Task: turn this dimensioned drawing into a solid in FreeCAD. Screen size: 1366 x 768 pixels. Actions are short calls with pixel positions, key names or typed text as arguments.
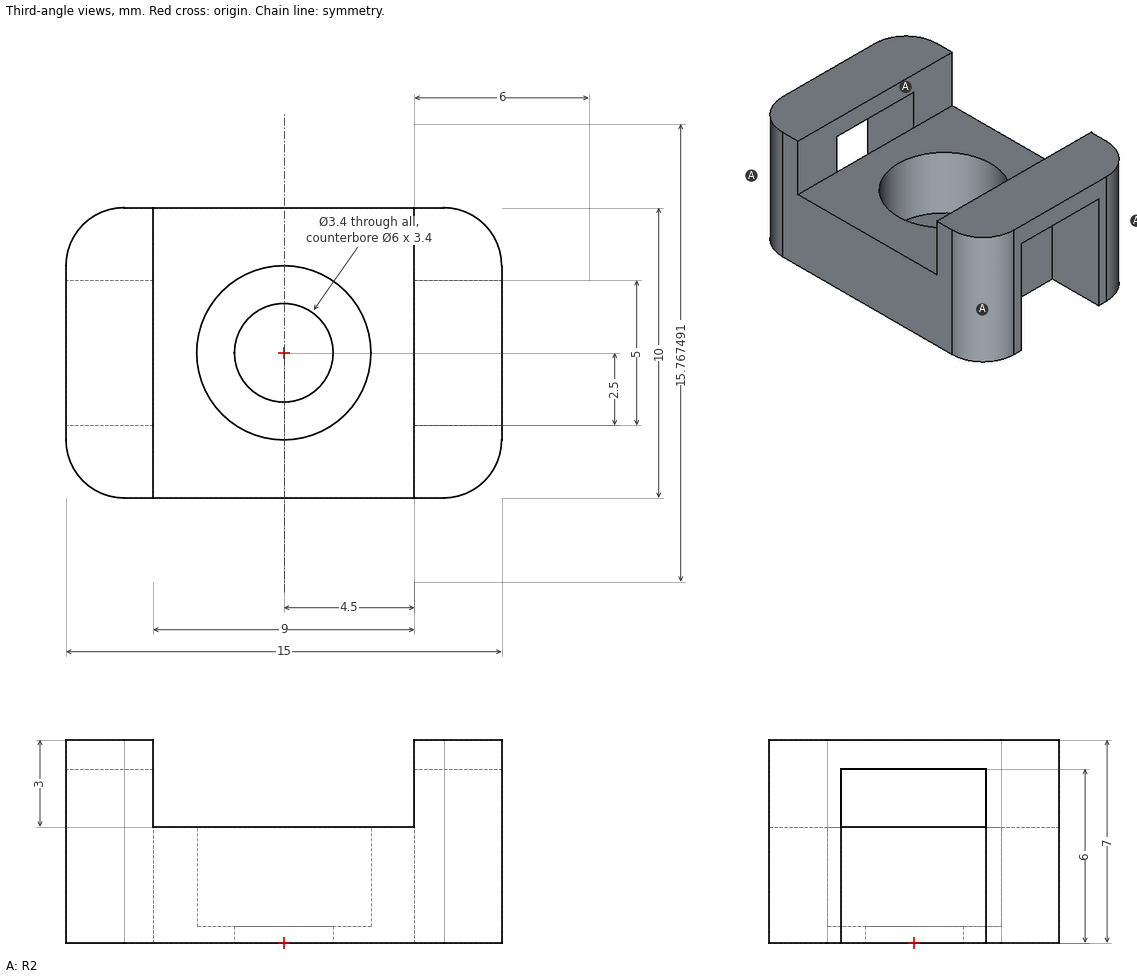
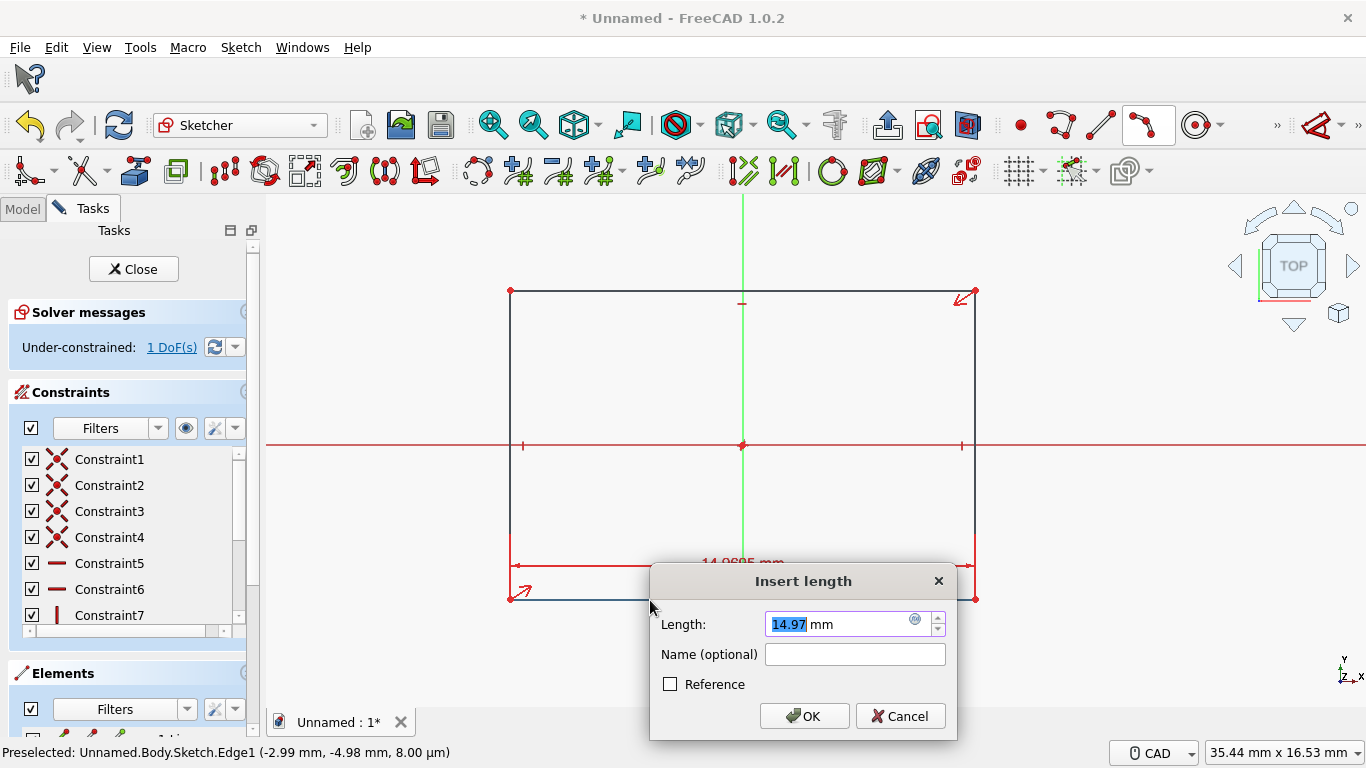
text(15)
key(Return)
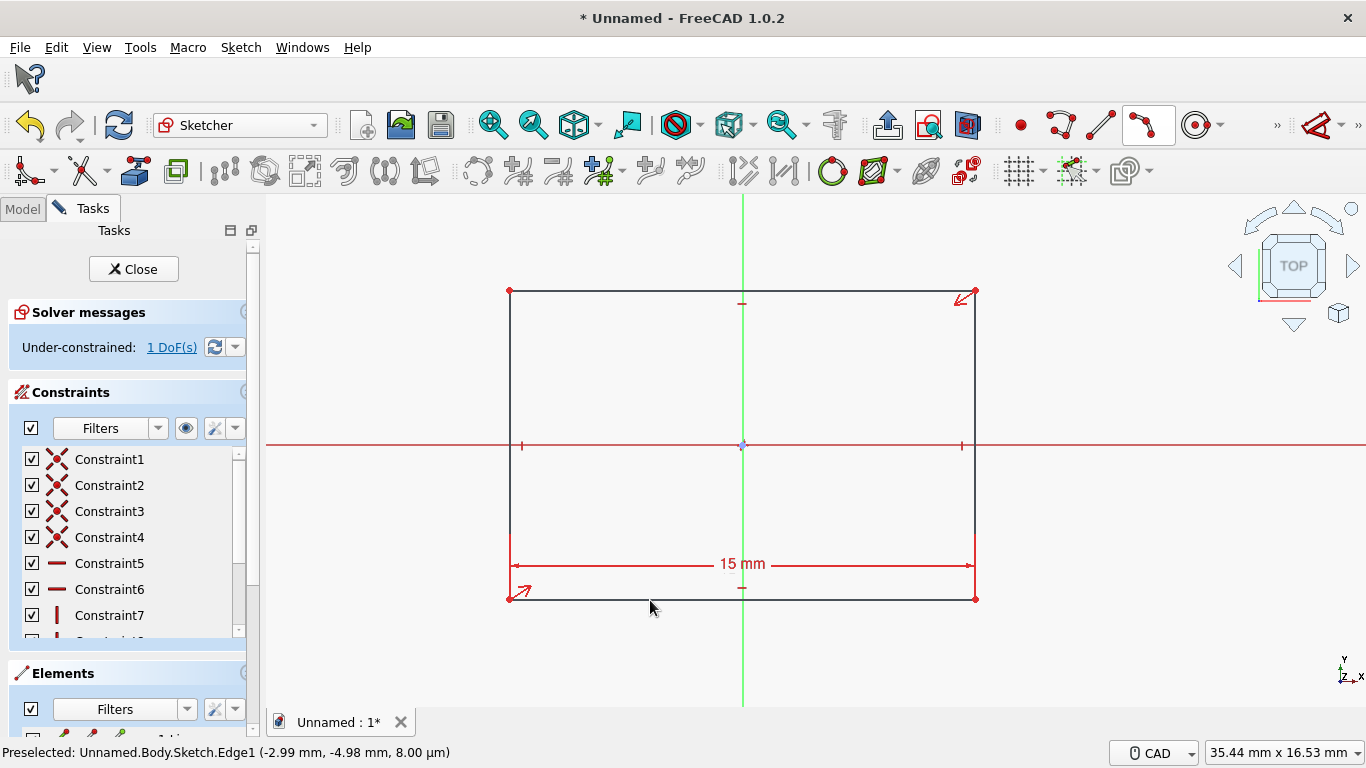
click(975, 507)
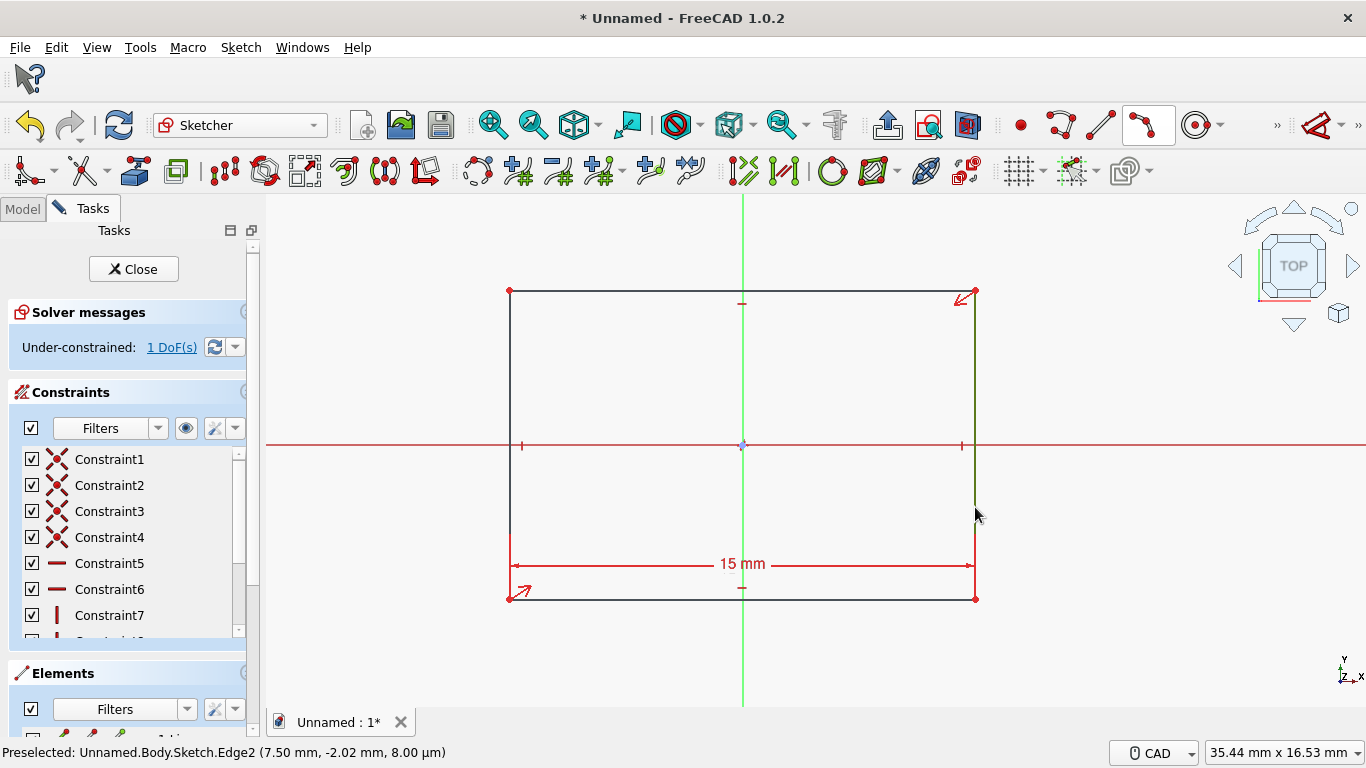
key(i)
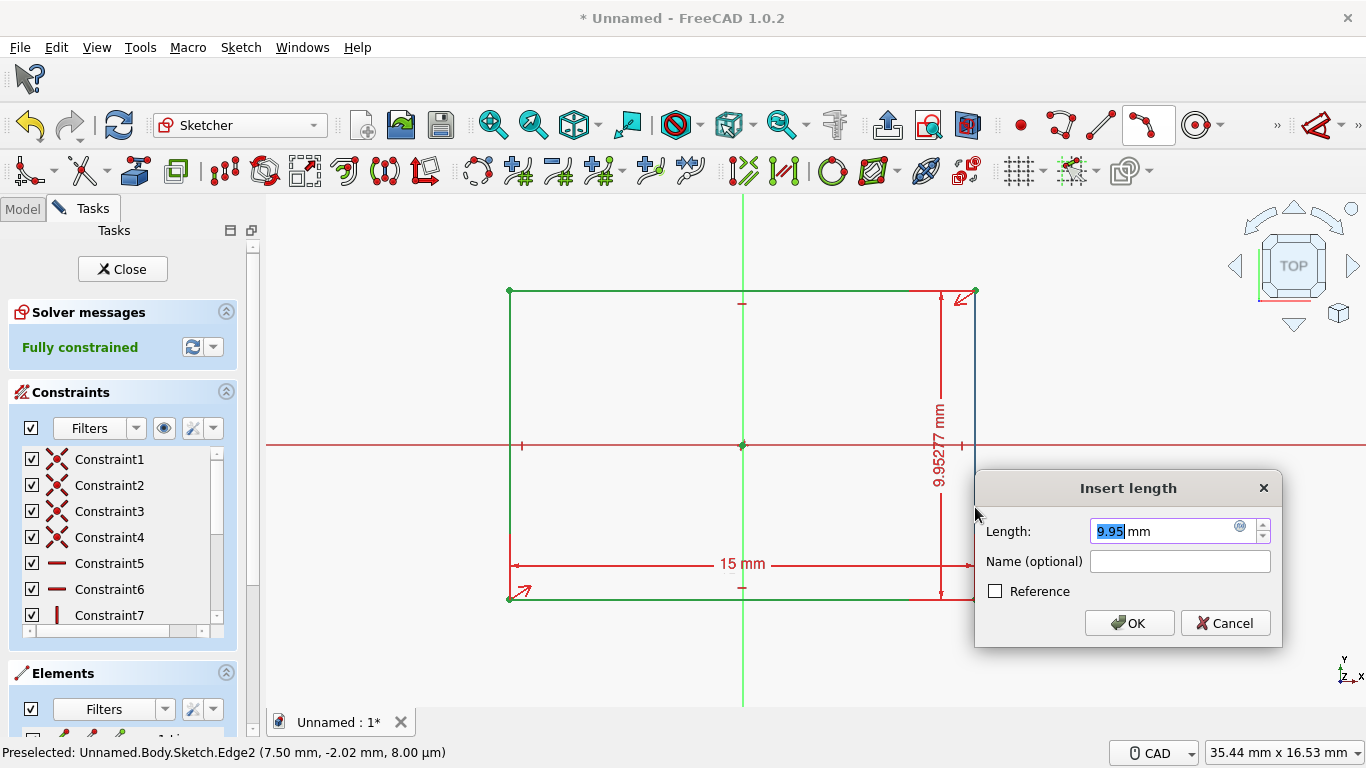
text(10)
key(Return)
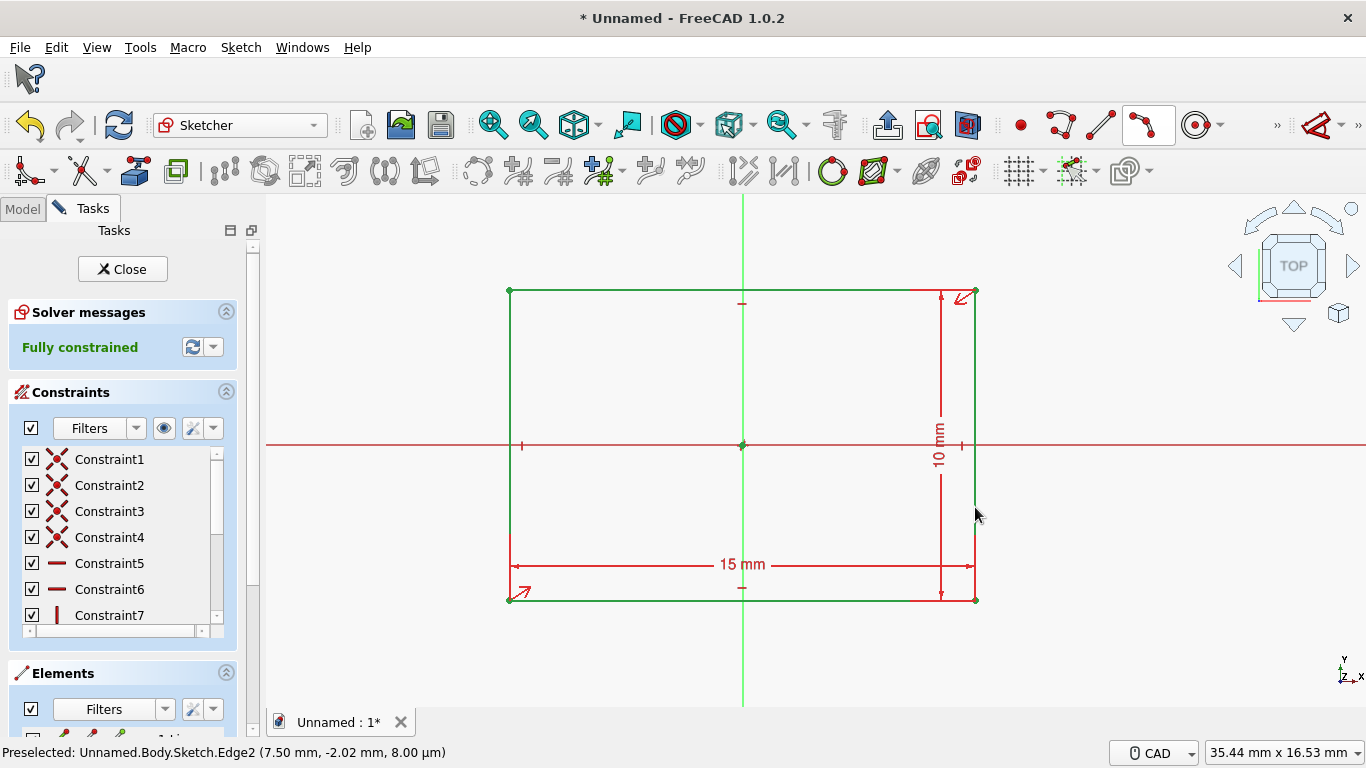
click(123, 269)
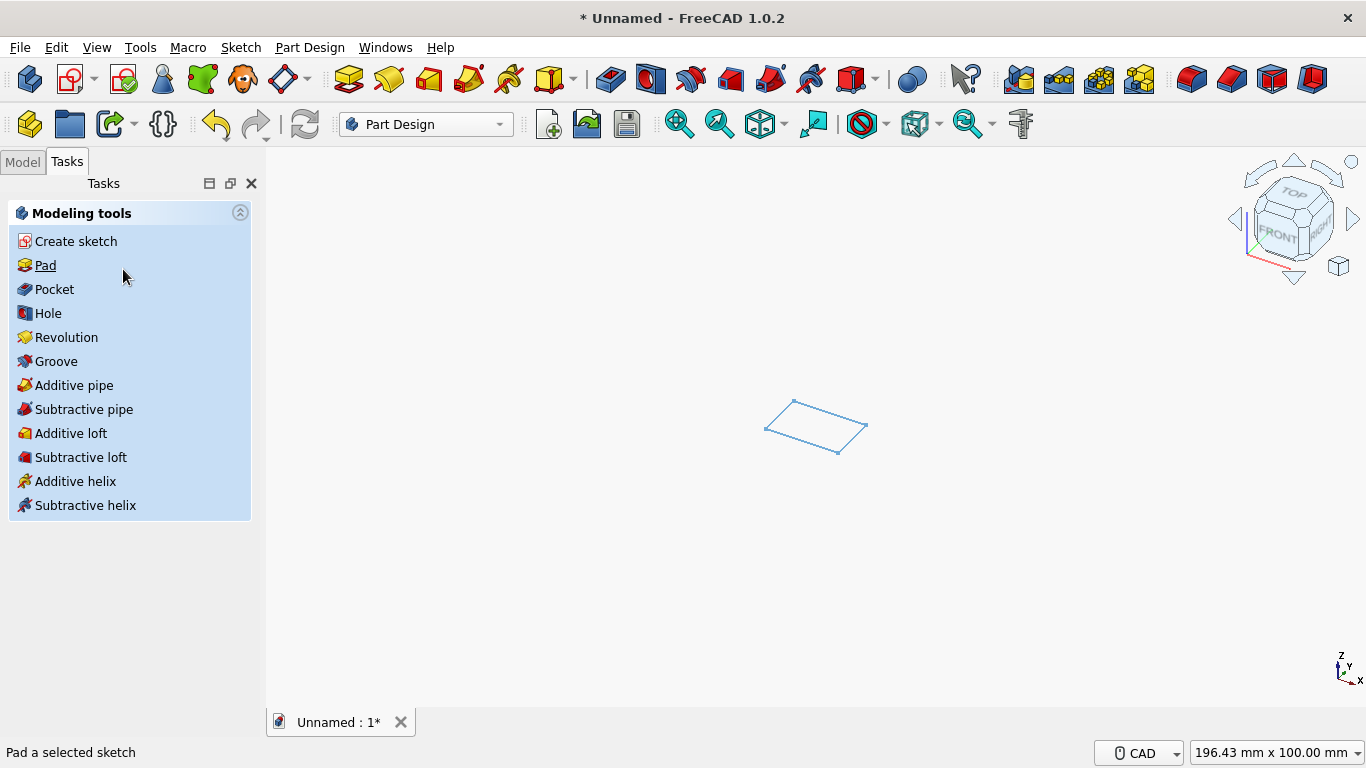
click(350, 80)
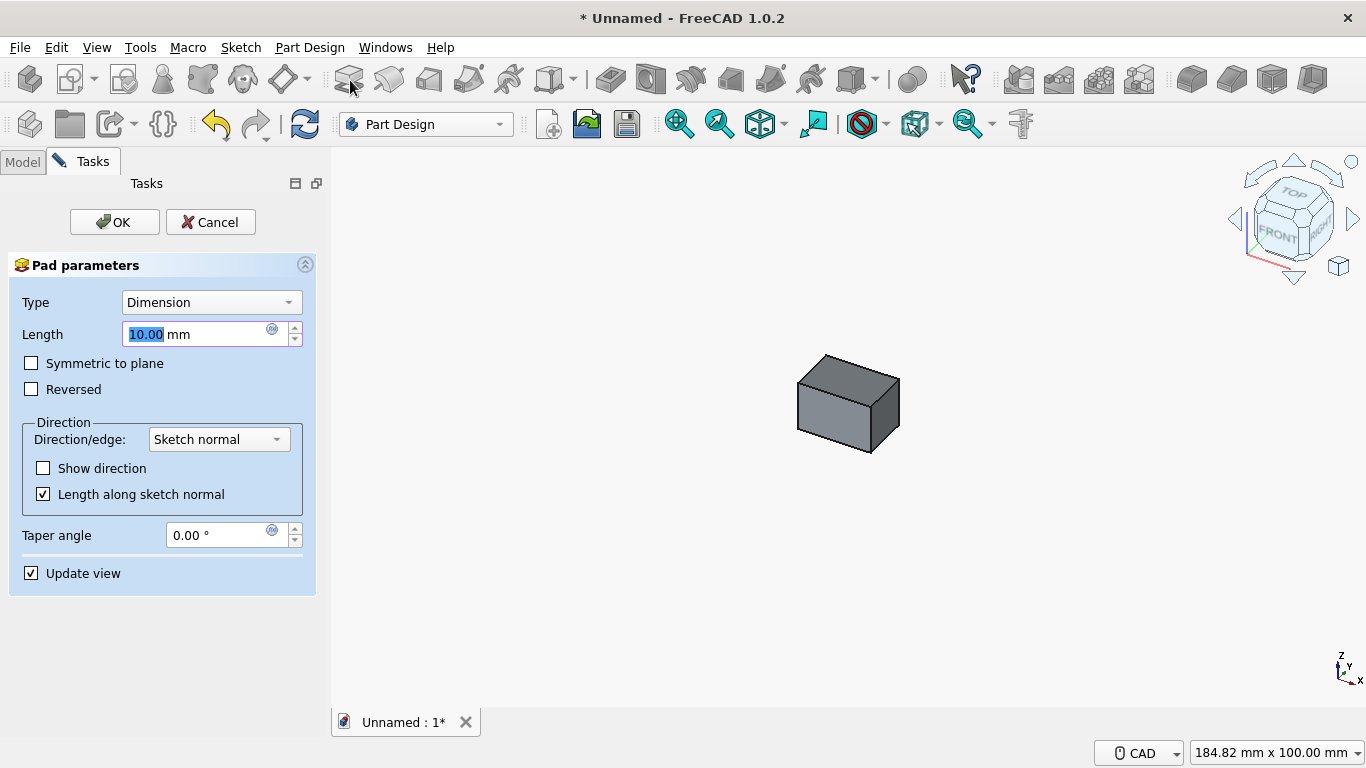
text(7)
key(Tab)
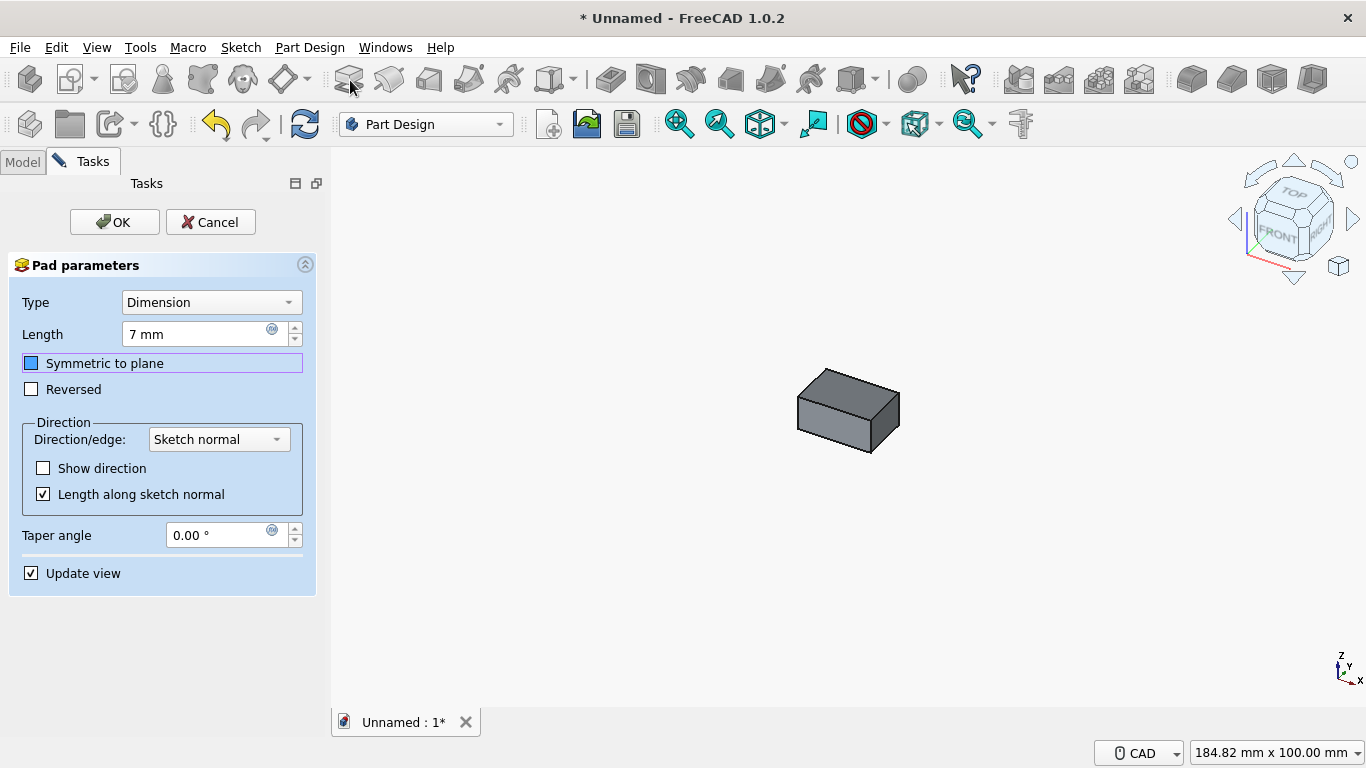
click(115, 222)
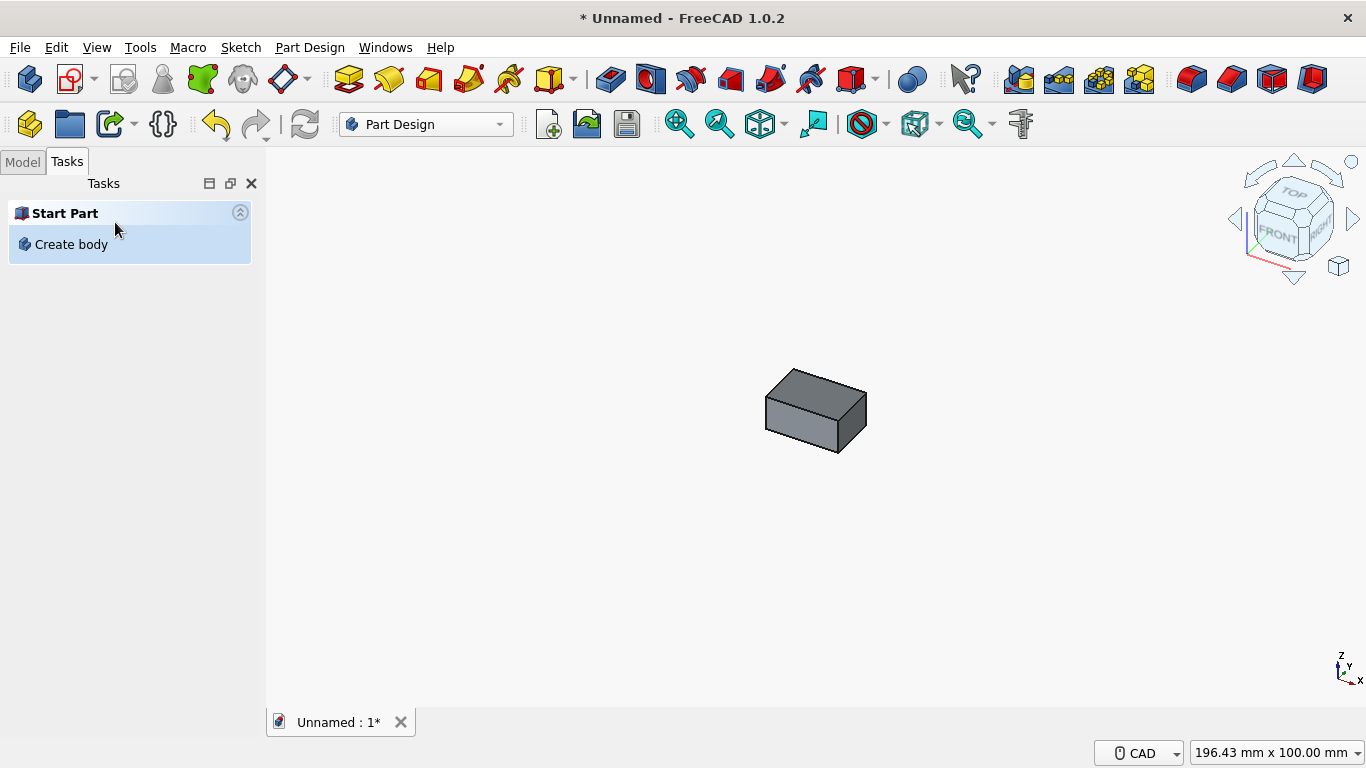
click(680, 124)